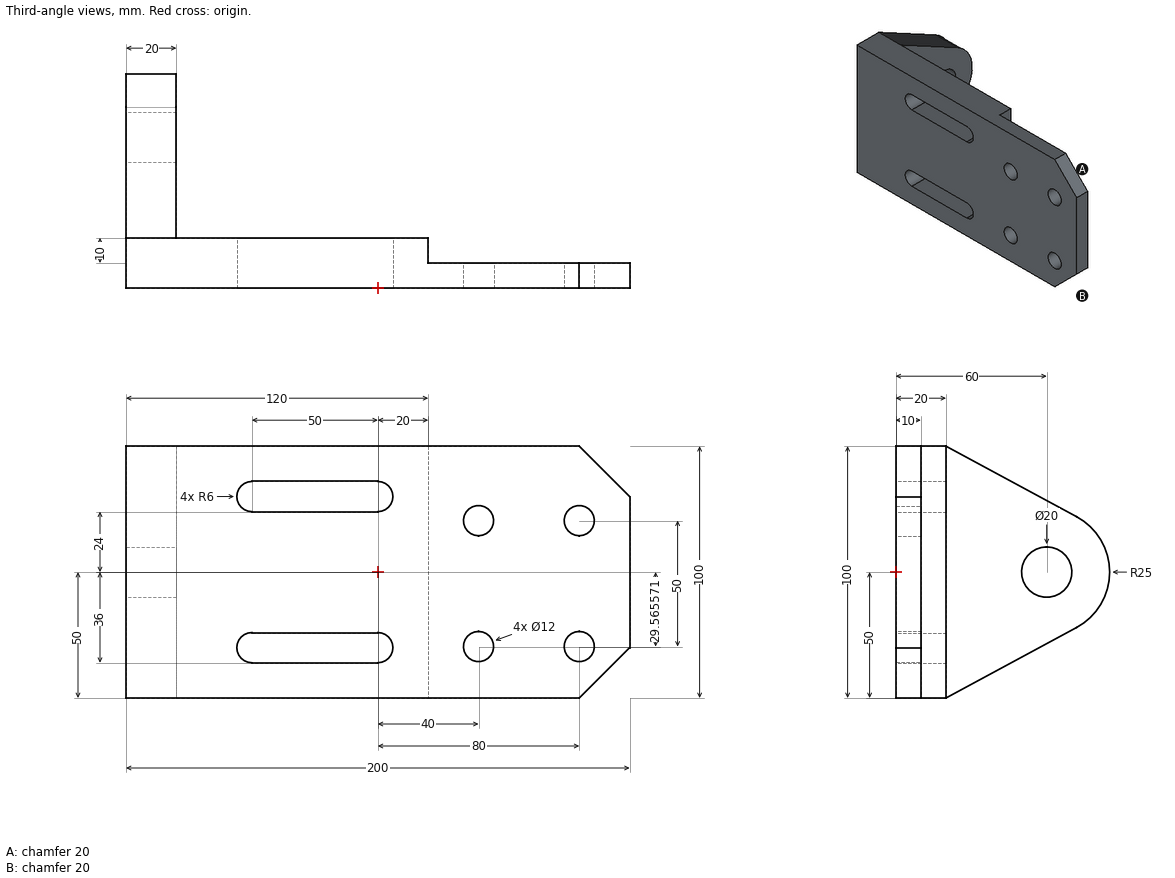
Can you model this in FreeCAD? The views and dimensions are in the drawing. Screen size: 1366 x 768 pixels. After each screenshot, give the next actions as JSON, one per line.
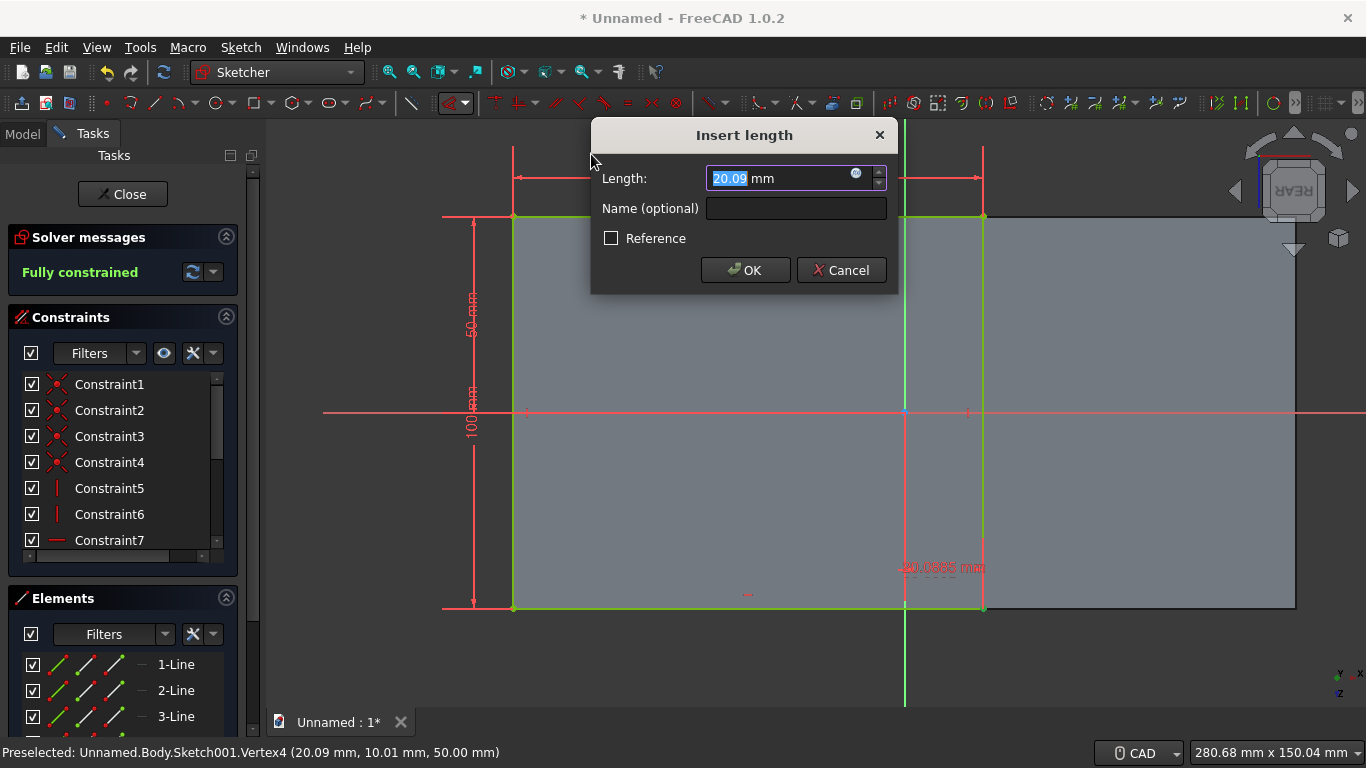
{"action": "type", "text": "20"}
{"action": "key", "text": "Return"}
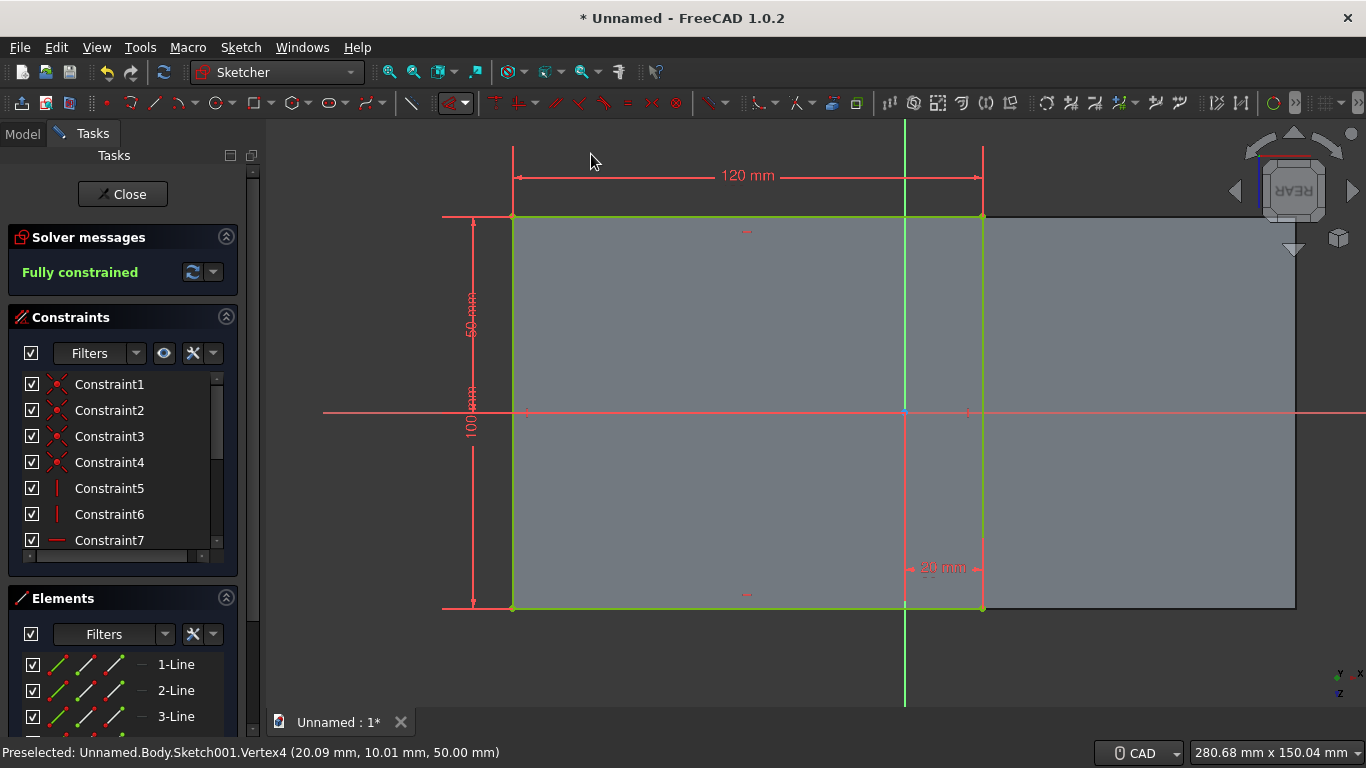
{"action": "left_click", "coordinate": [123, 194]}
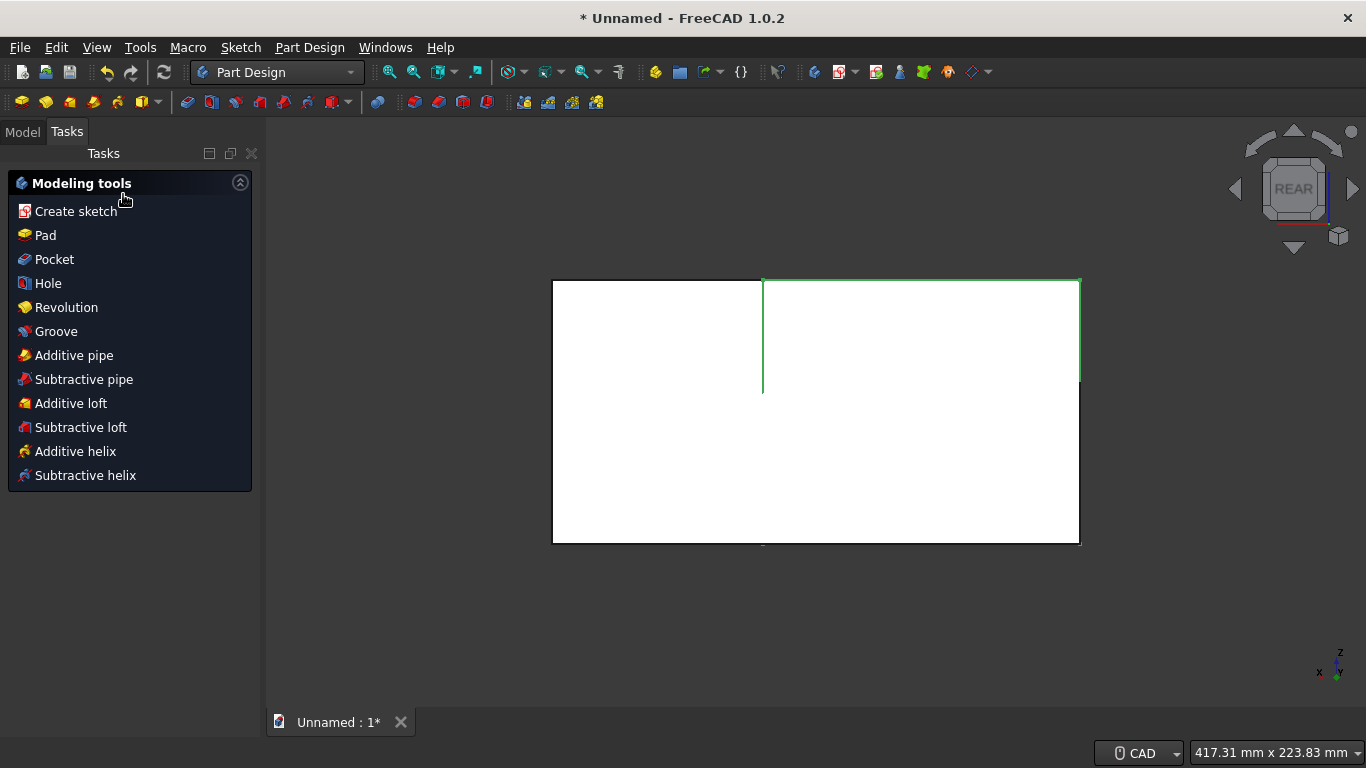
{"action": "left_click", "coordinate": [22, 102]}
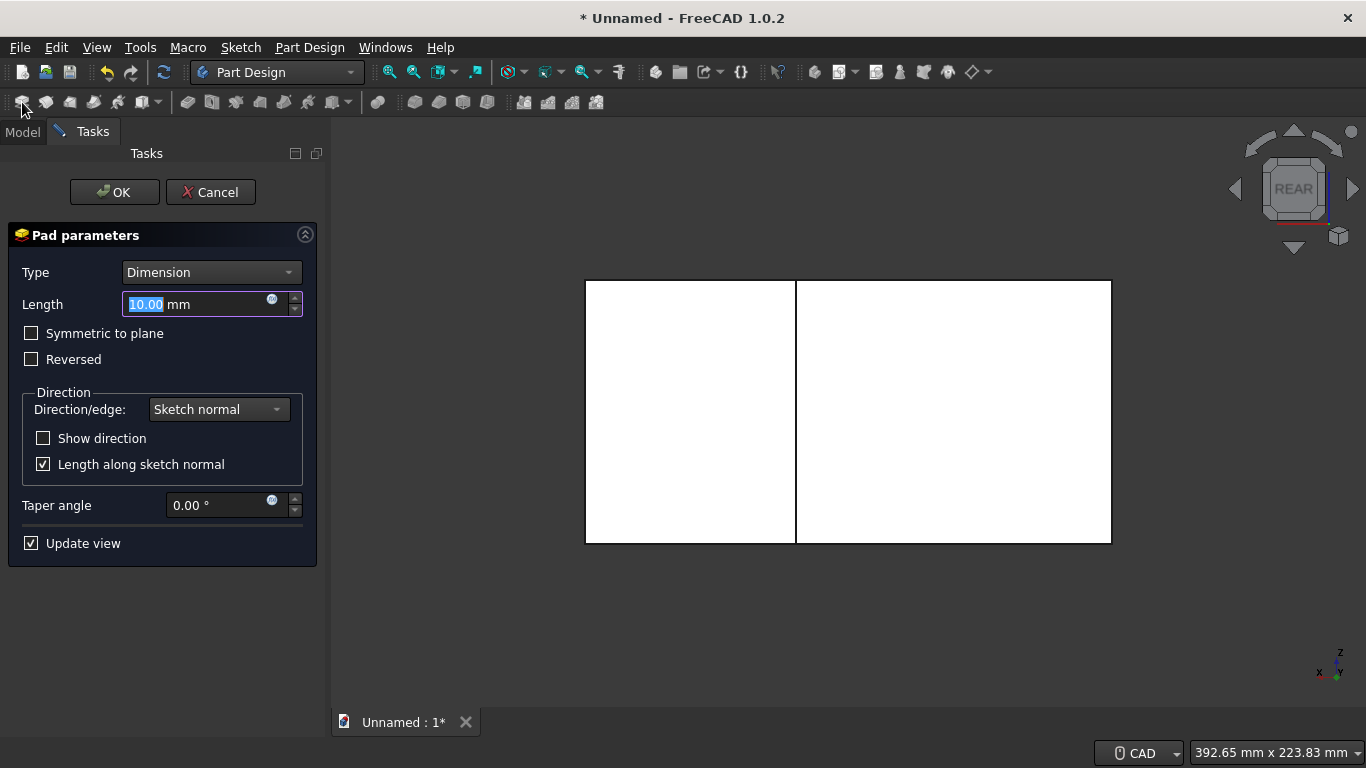
{"action": "type", "text": "10"}
{"action": "key", "text": "Tab"}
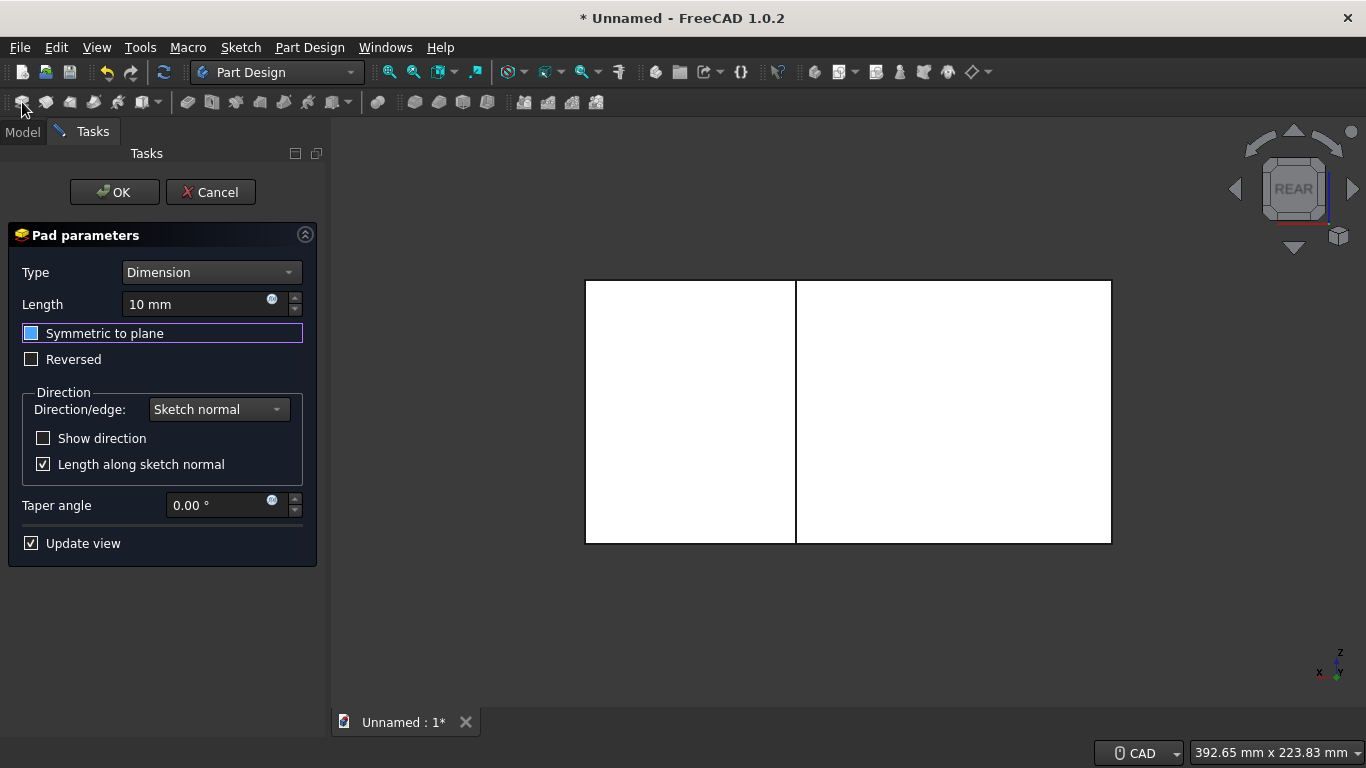
{"action": "left_click", "coordinate": [115, 192]}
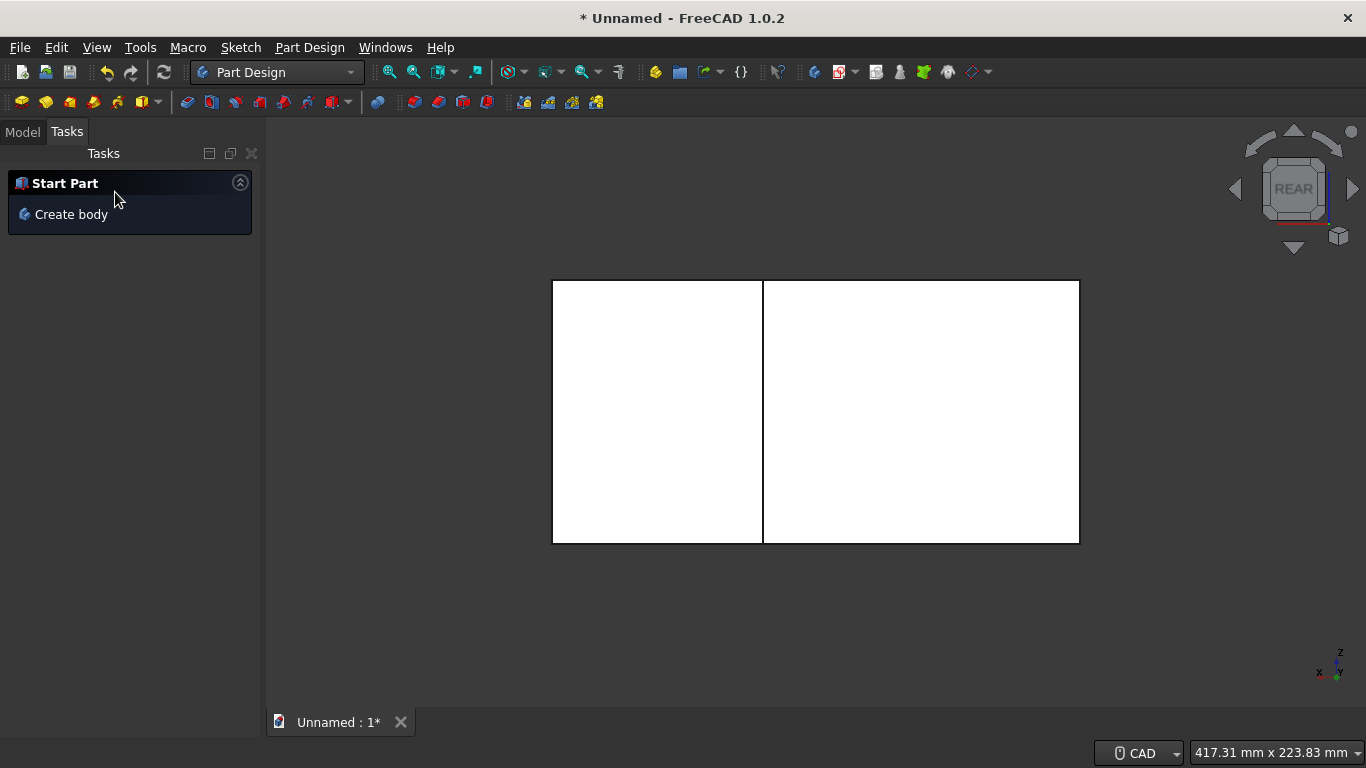
{"action": "key", "text": "0"}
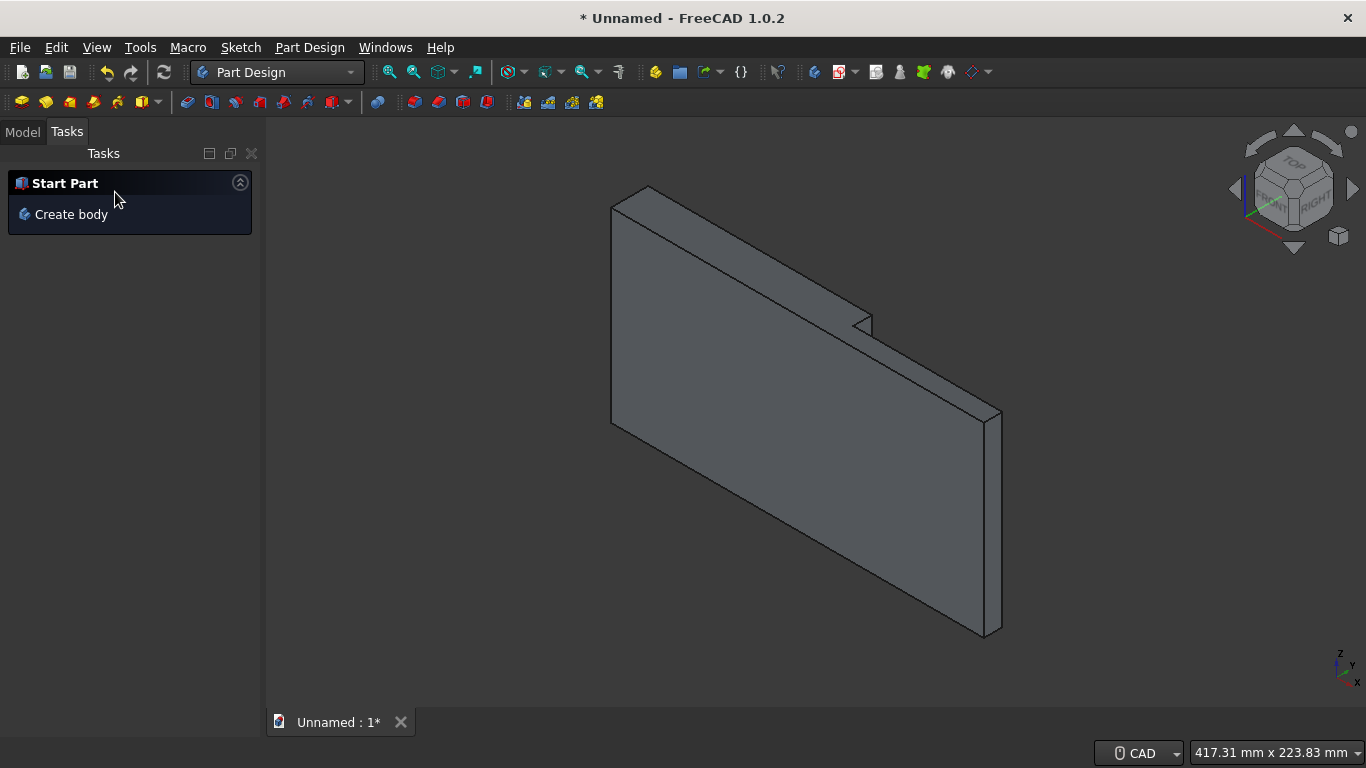
{"action": "left_click", "coordinate": [993, 416]}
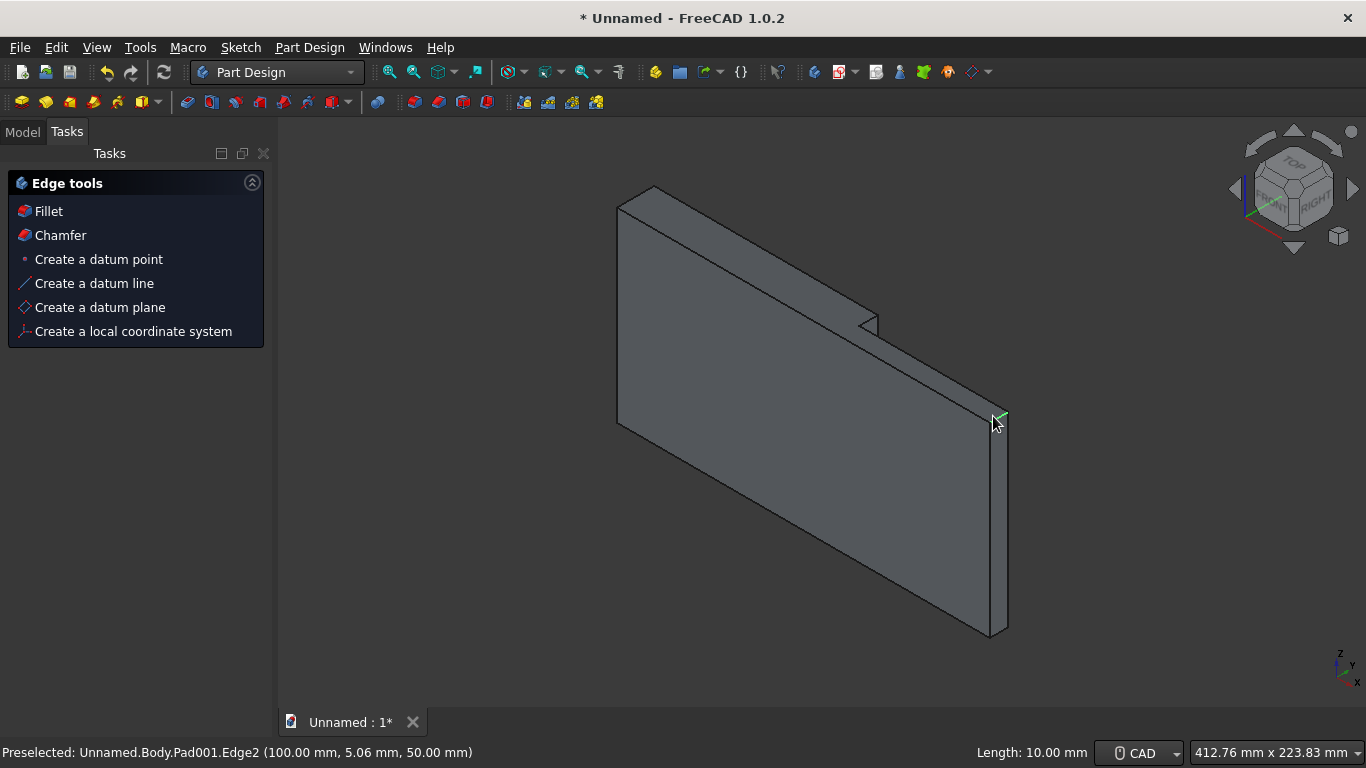
{"action": "left_click", "coordinate": [440, 102]}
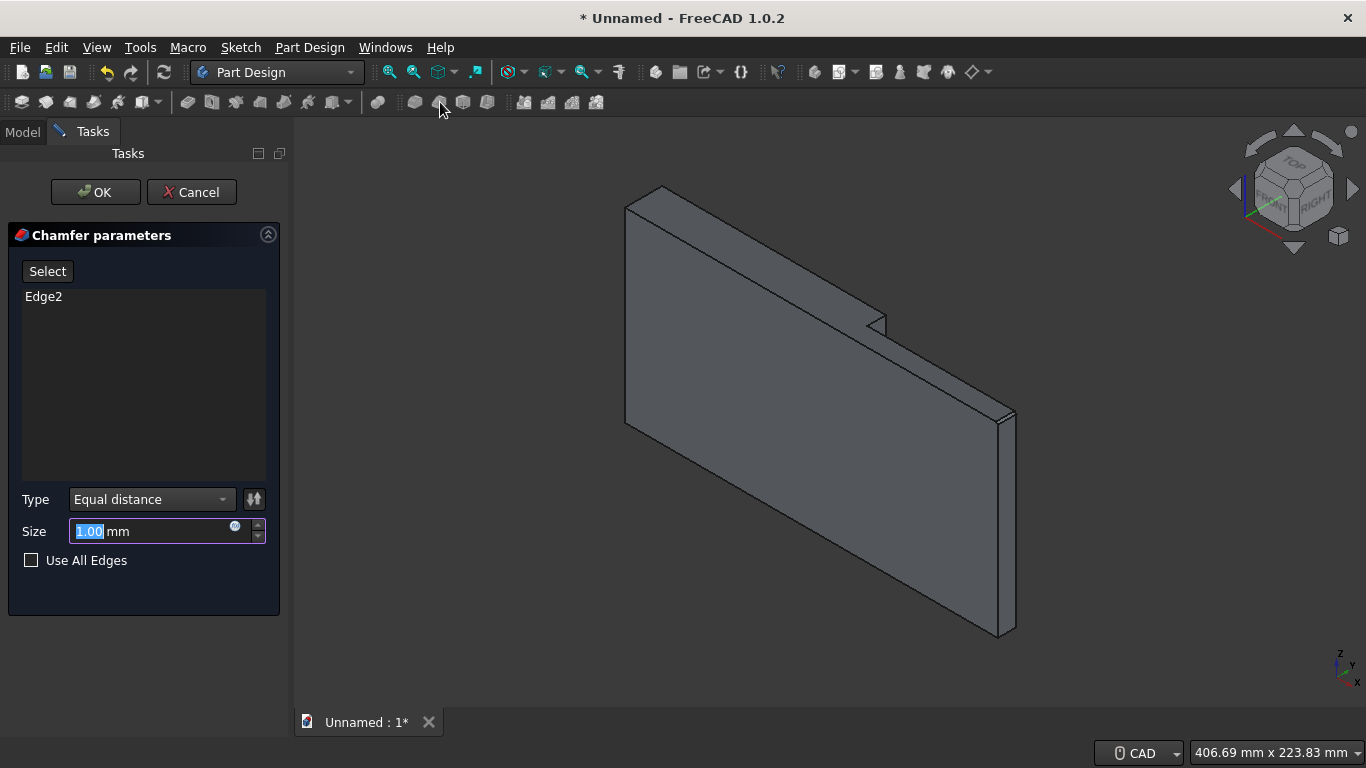
{"action": "type", "text": "20"}
{"action": "key", "text": "Tab"}